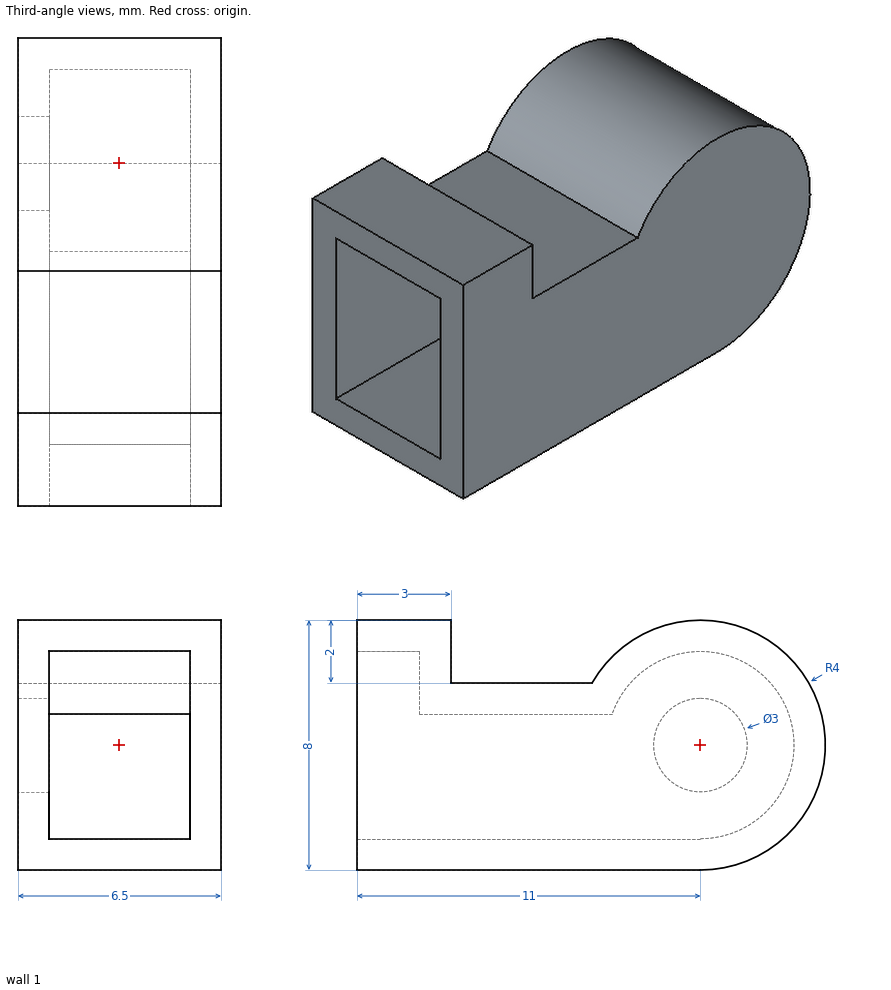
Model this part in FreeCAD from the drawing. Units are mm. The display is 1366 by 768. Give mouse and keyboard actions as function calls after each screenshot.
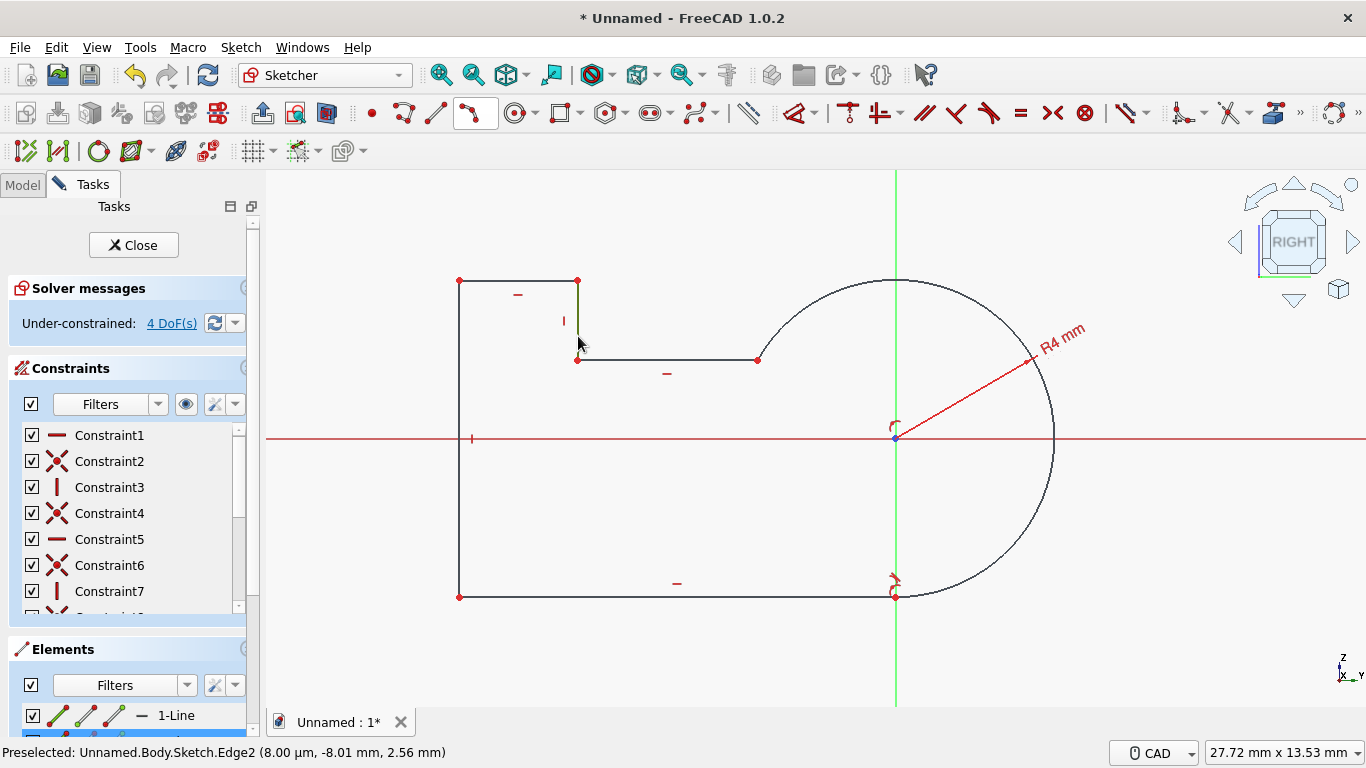
key(i)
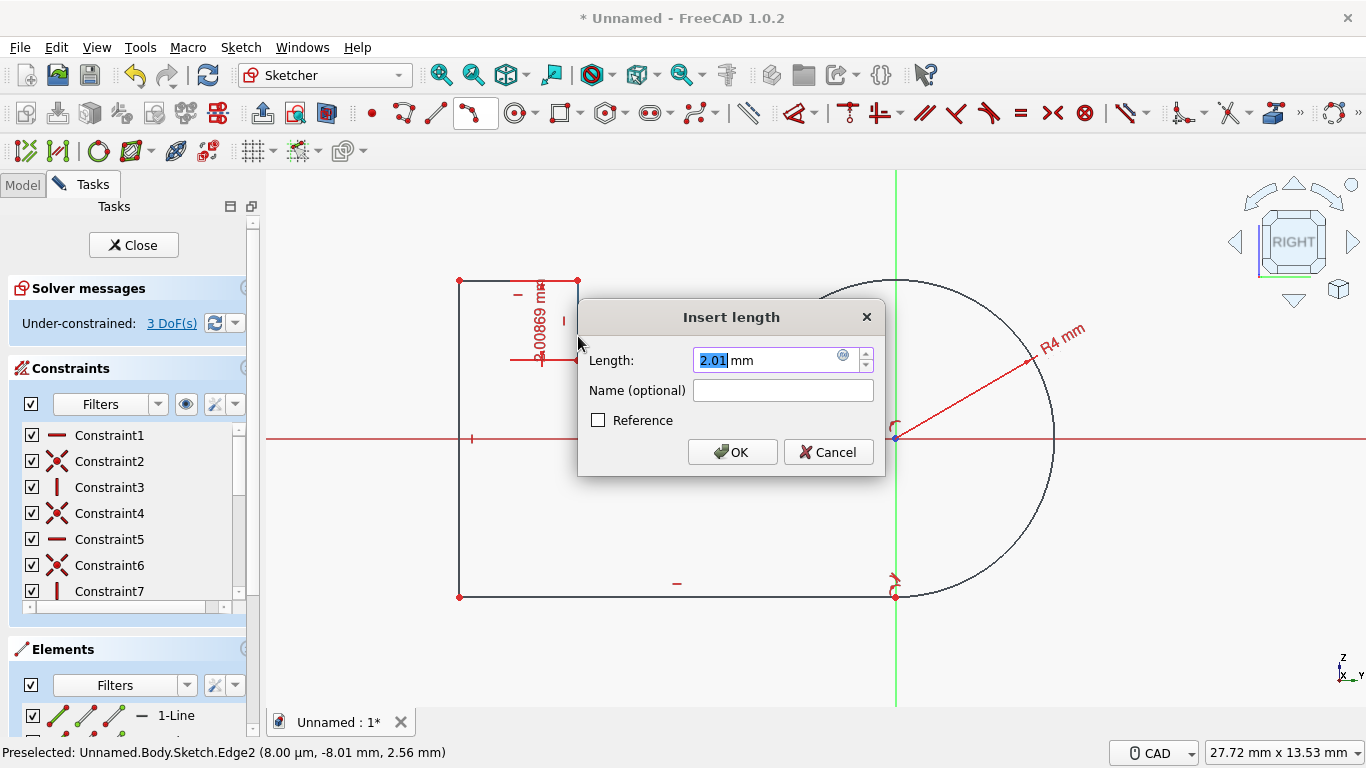
text(2)
key(Return)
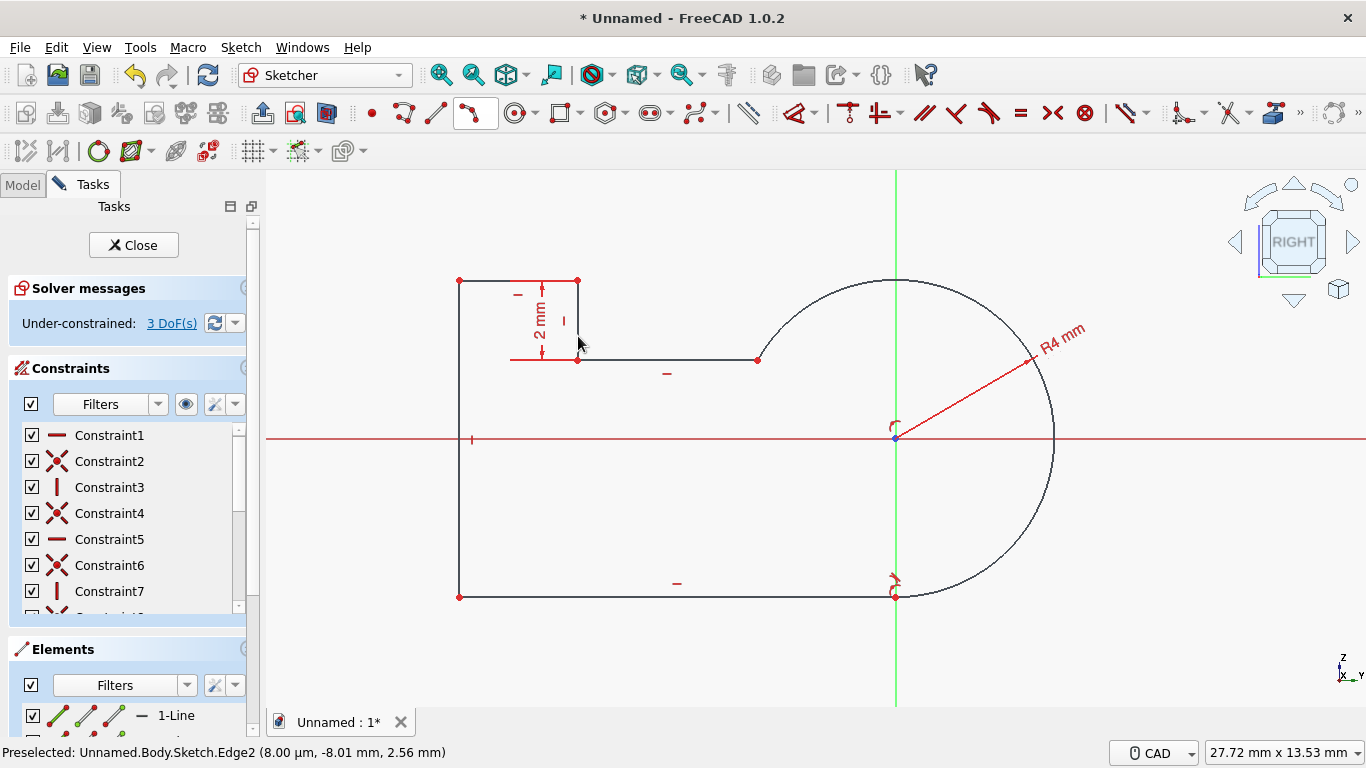
click(542, 281)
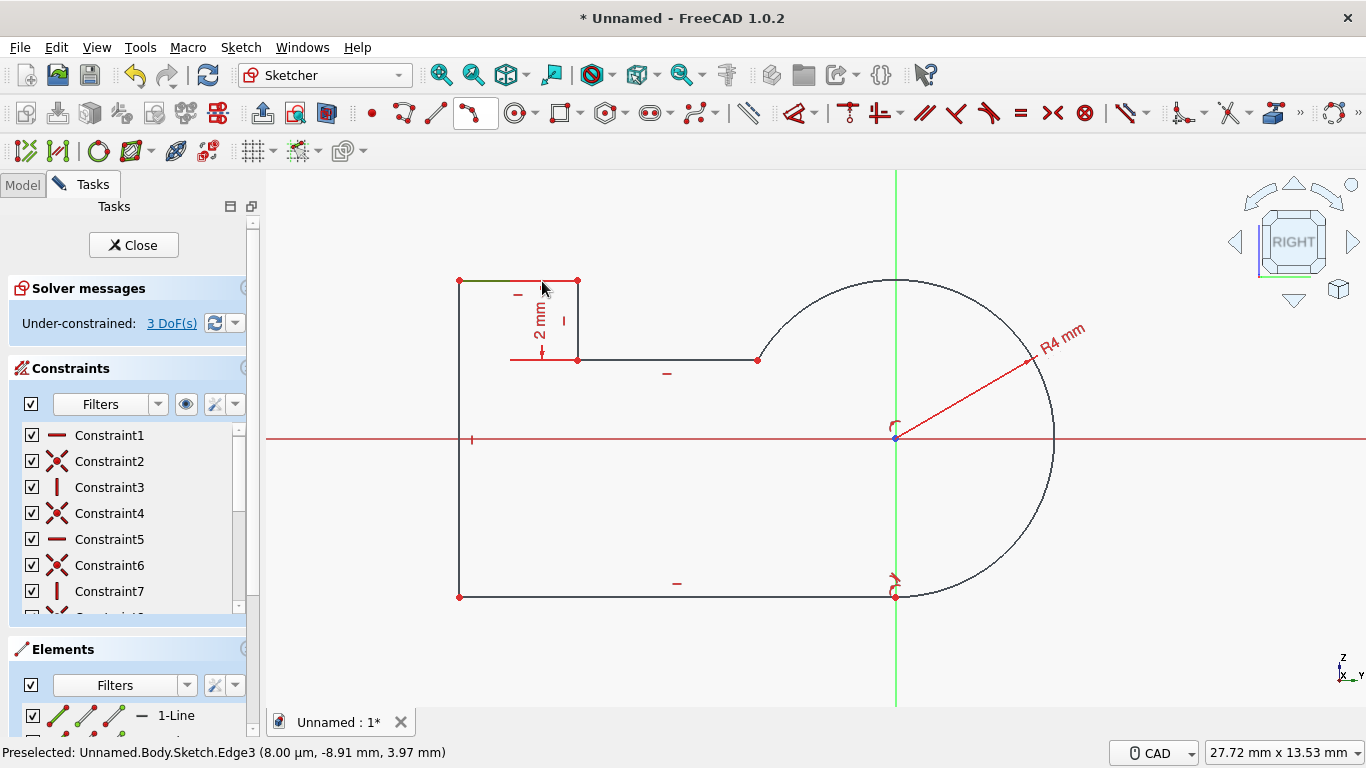
key(l)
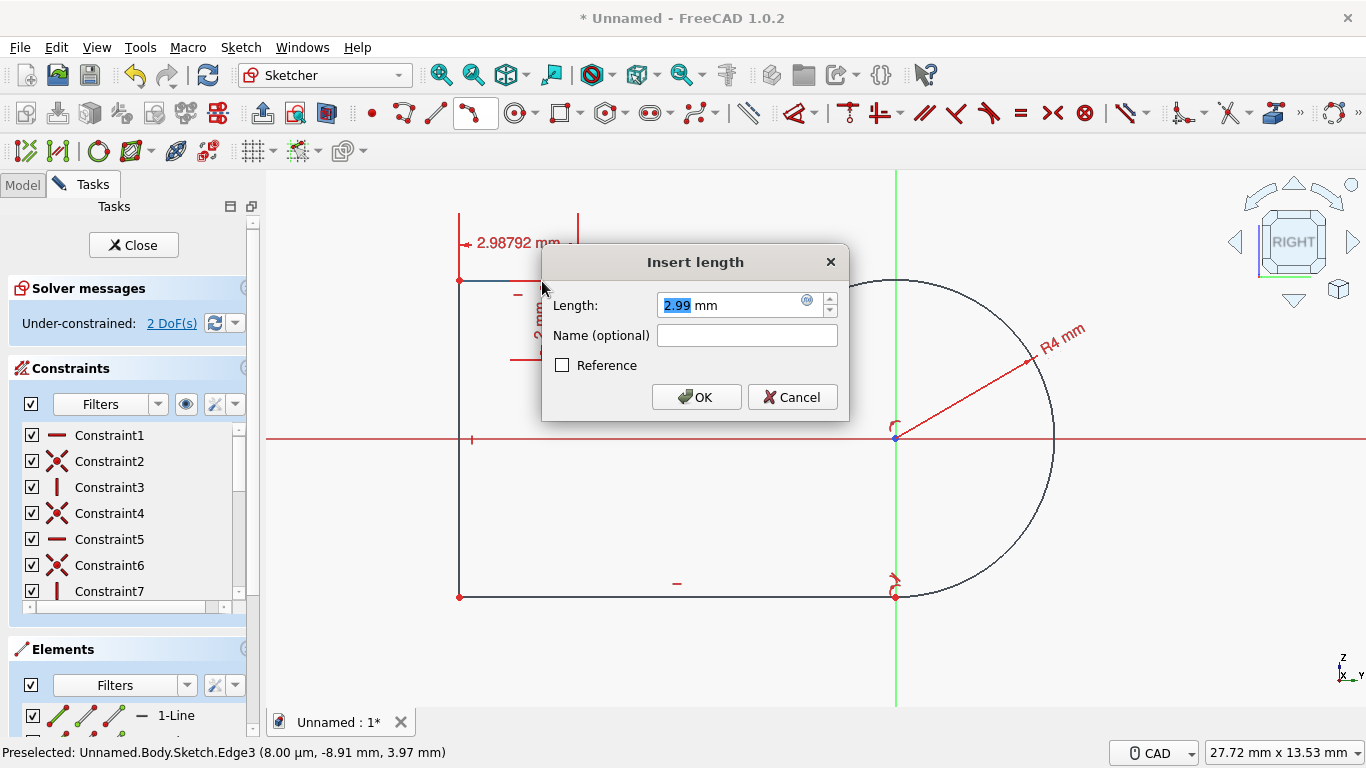
text(3)
key(Return)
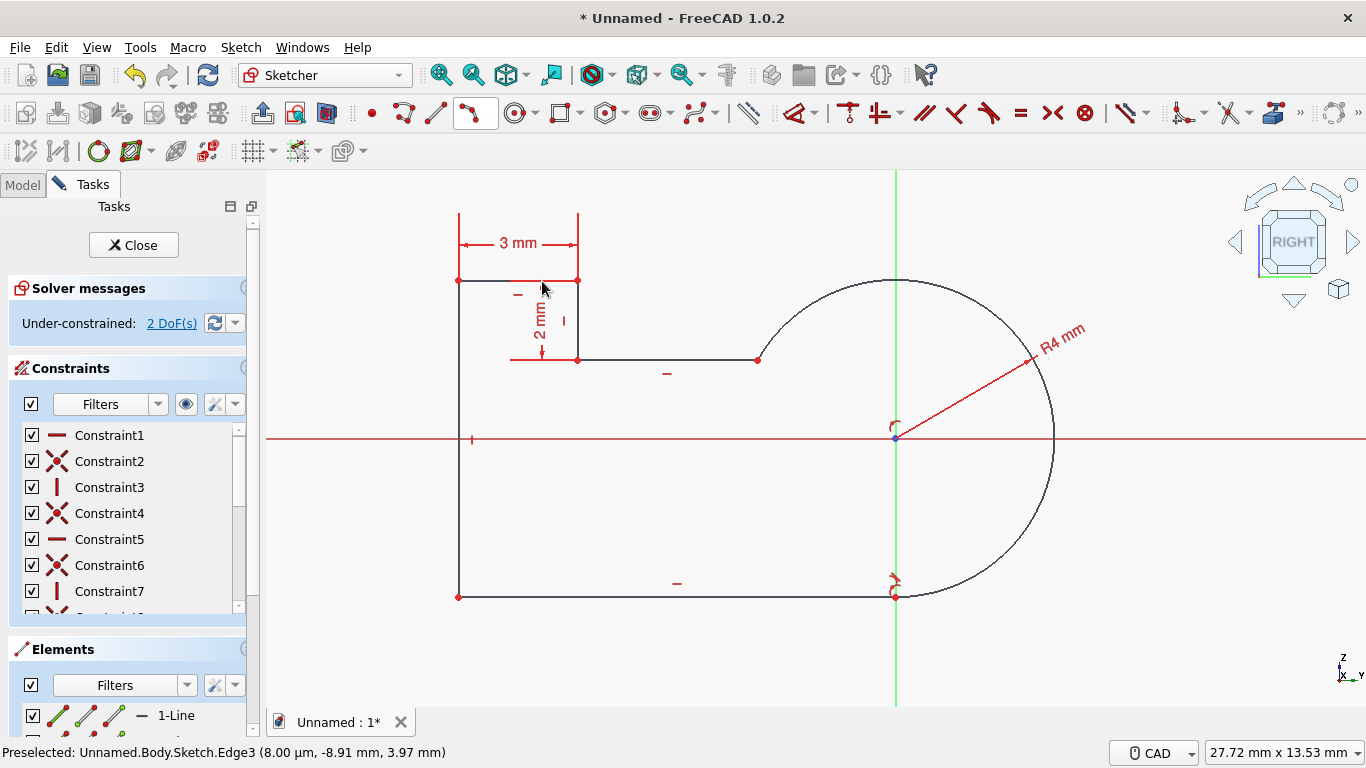
click(459, 376)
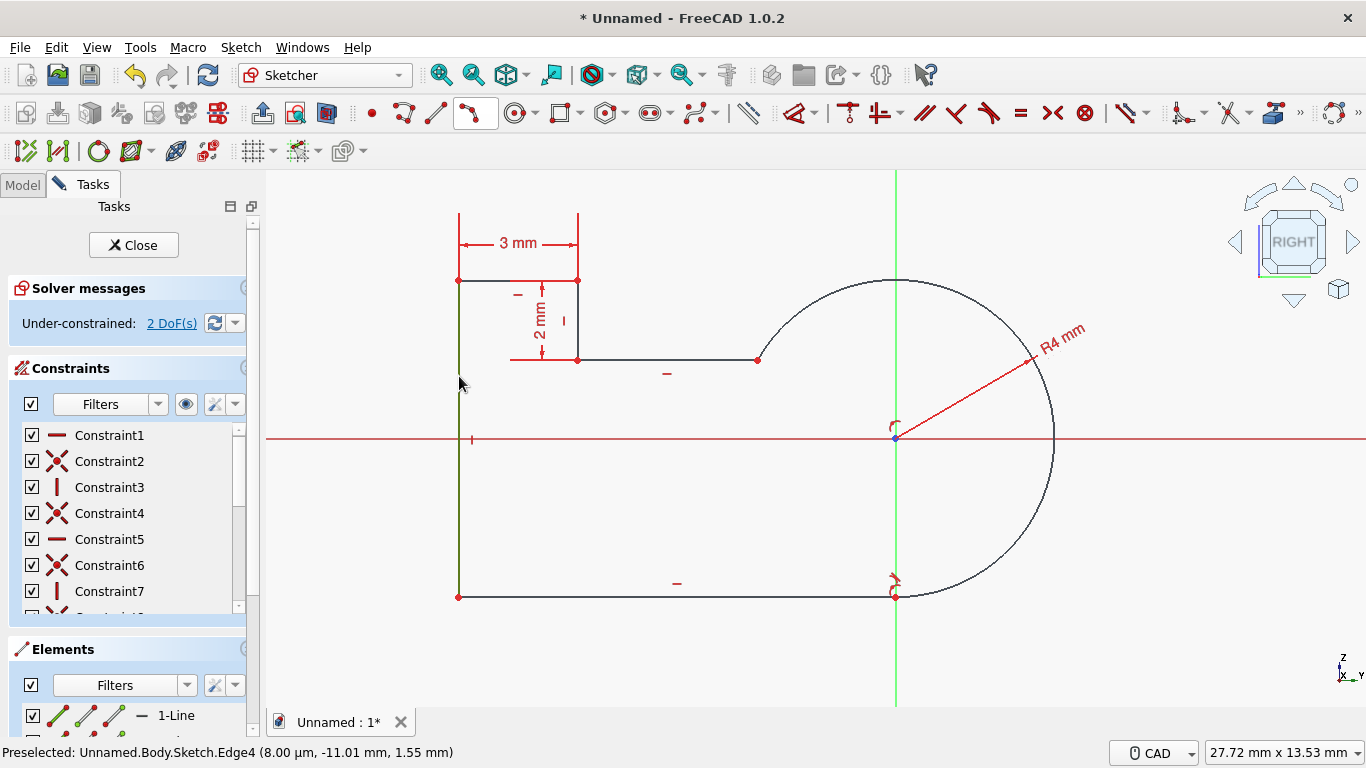
key(i)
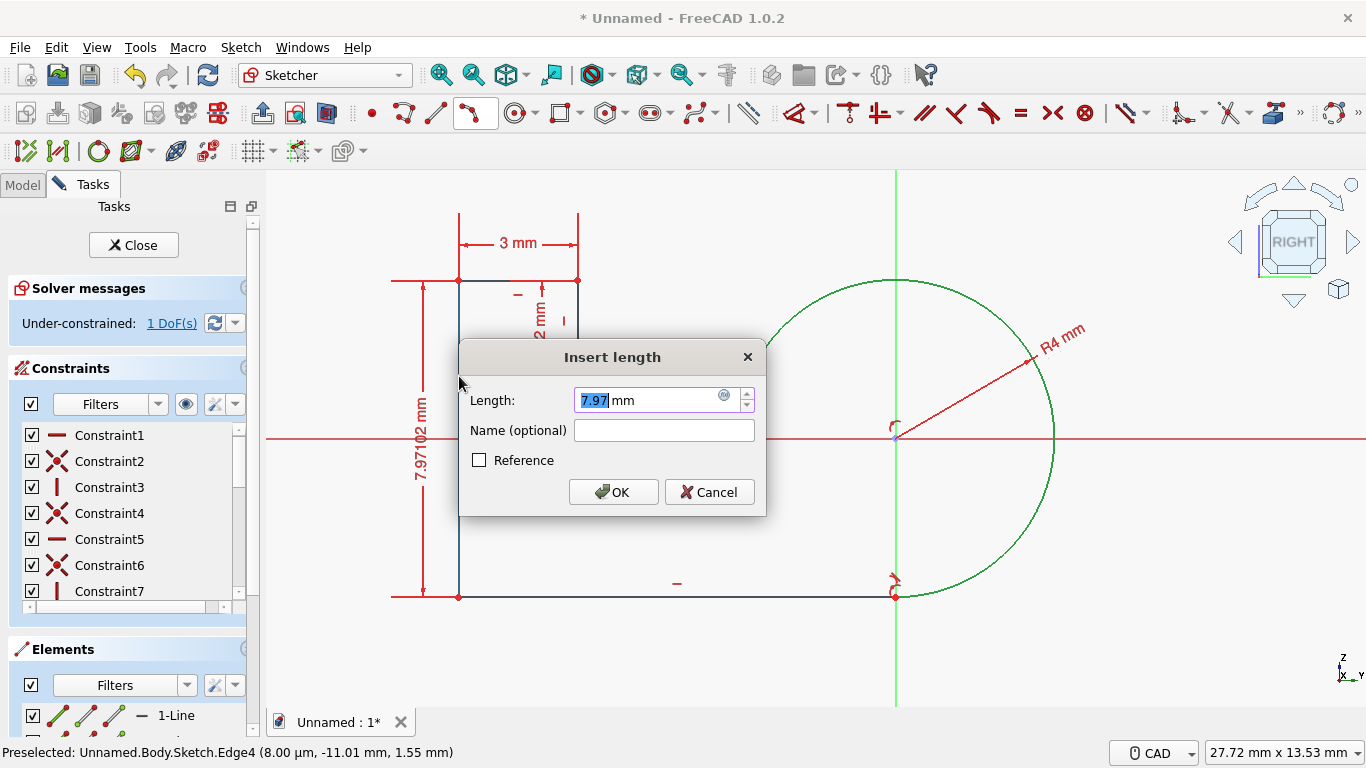
text(8)
key(Return)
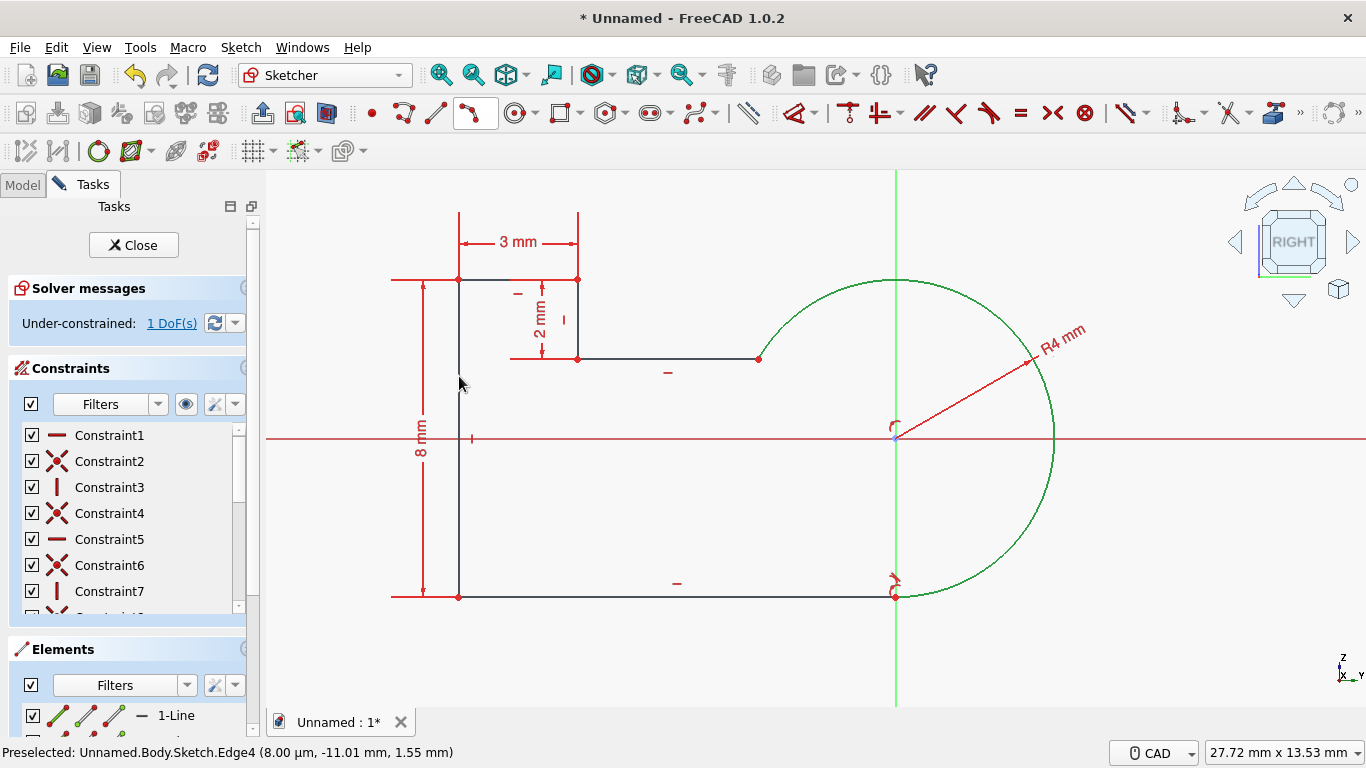
click(590, 597)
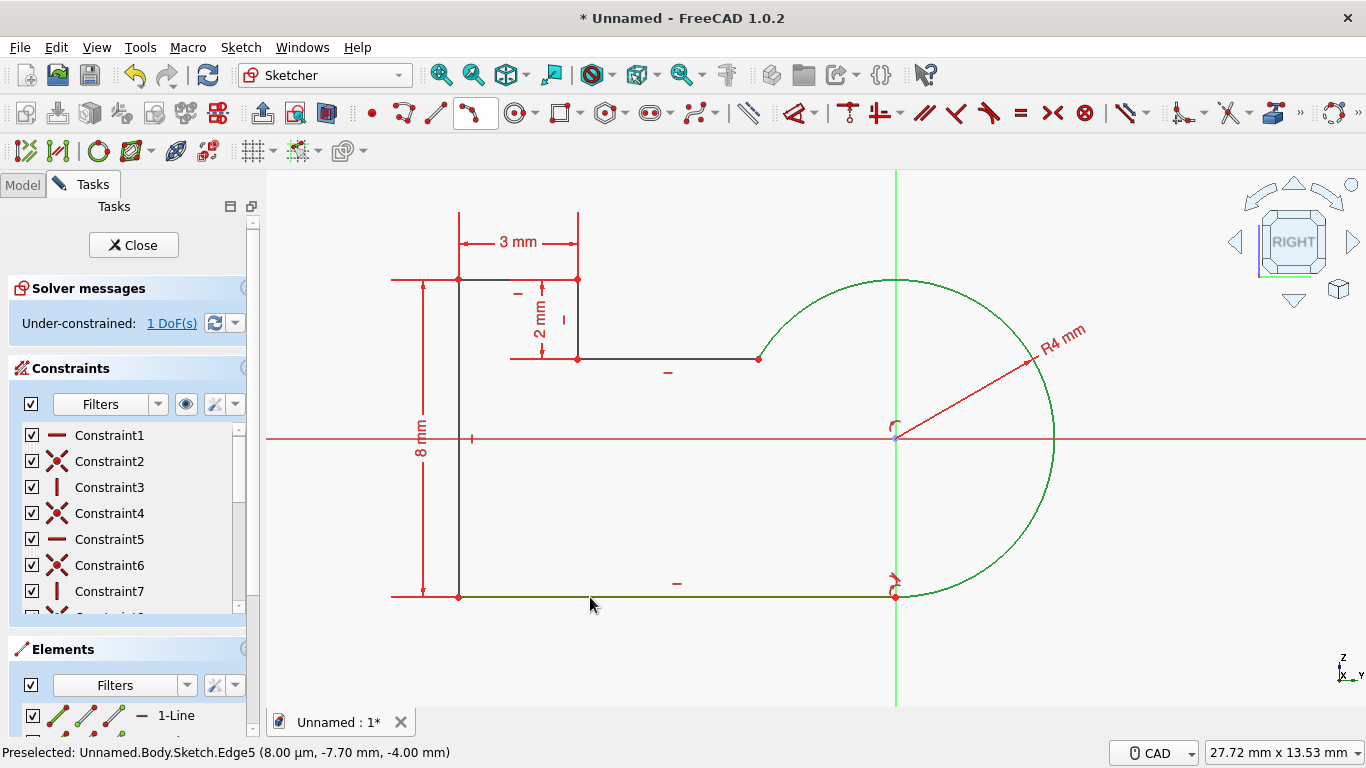
key(l)